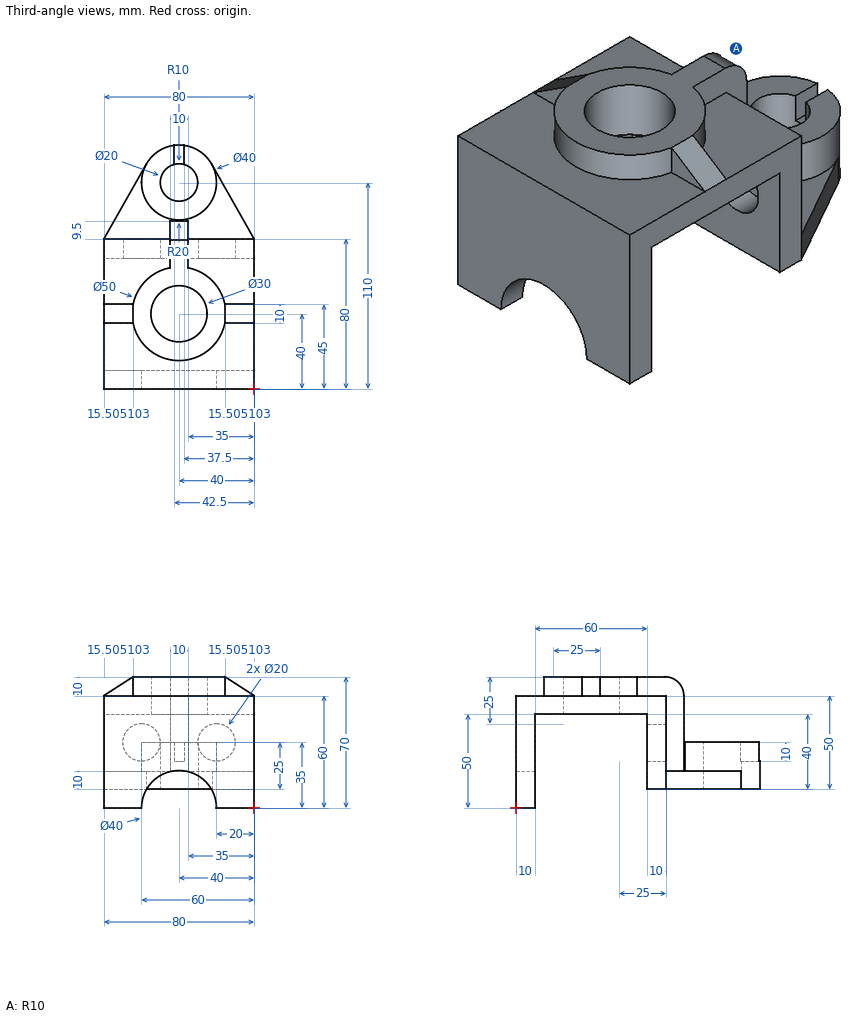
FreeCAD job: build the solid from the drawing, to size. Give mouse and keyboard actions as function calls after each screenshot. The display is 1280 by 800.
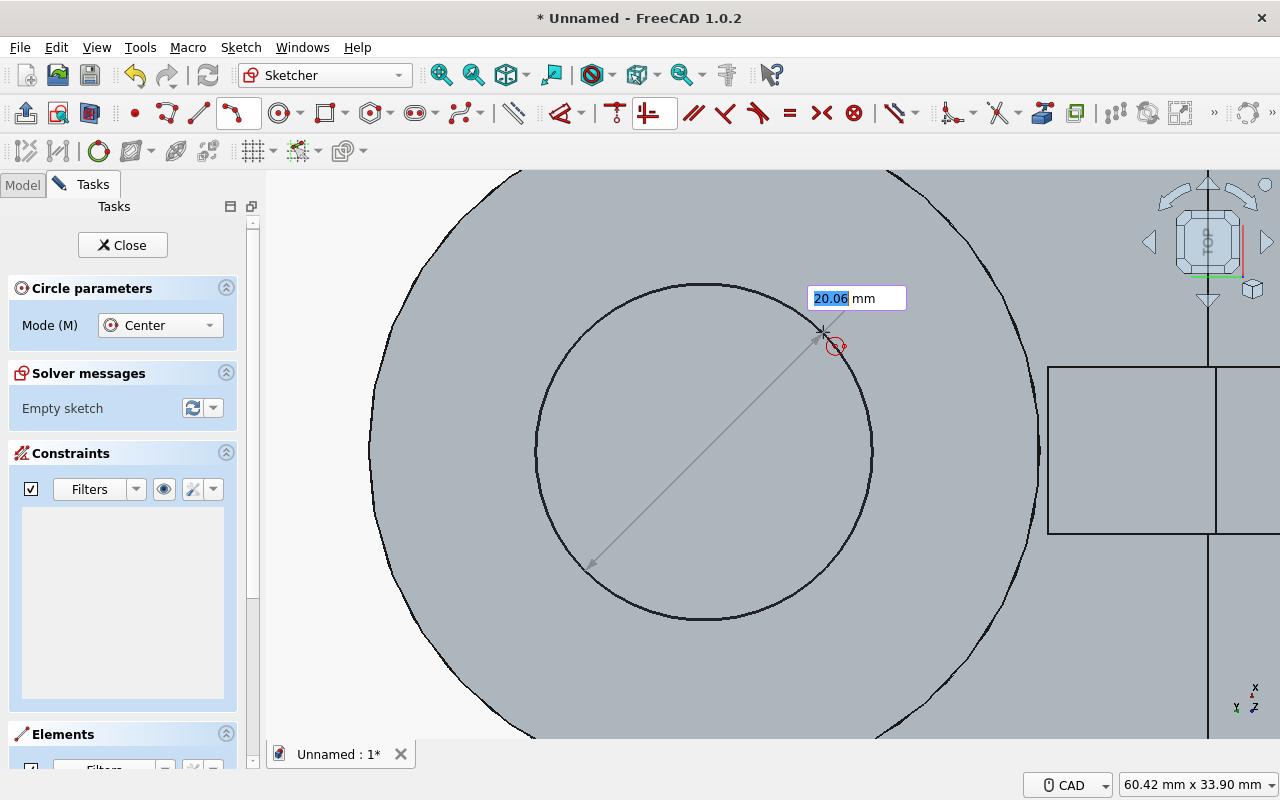
text(20)
key(Return)
key(Escape)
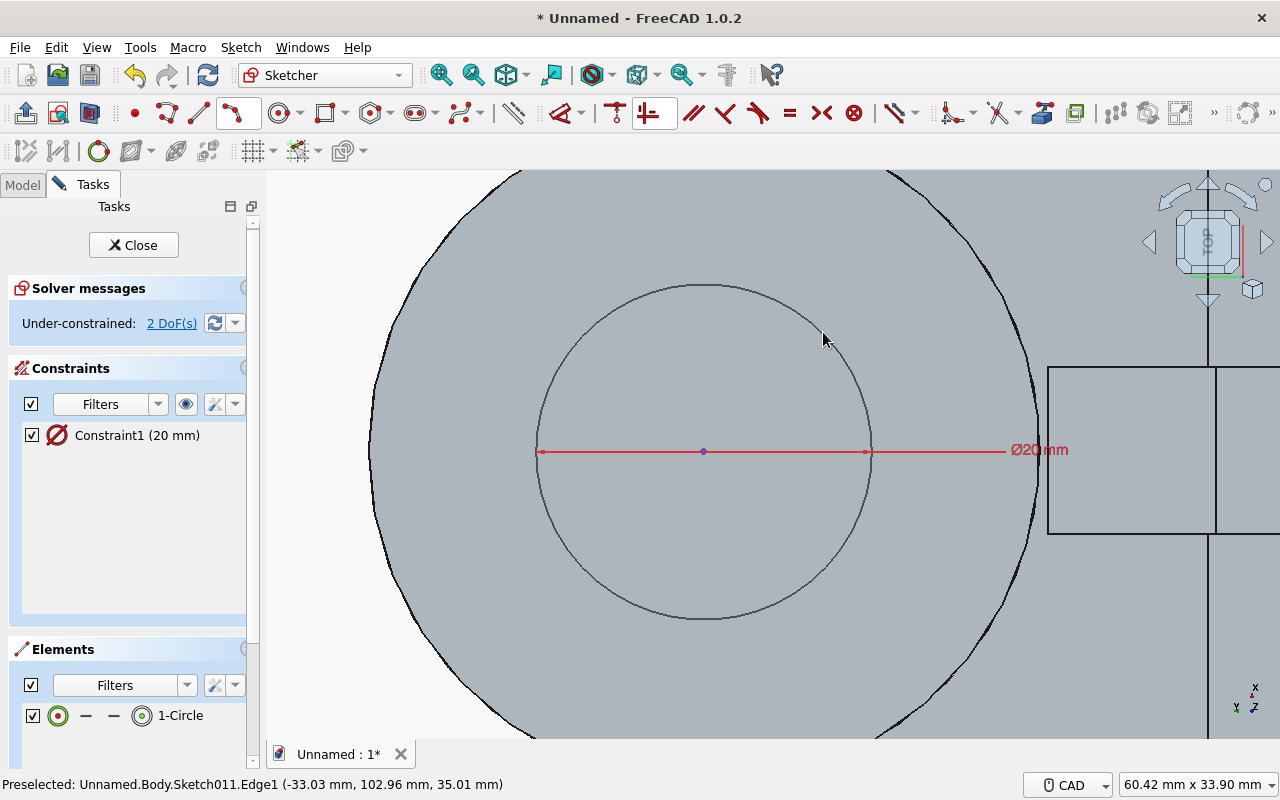
click(560, 114)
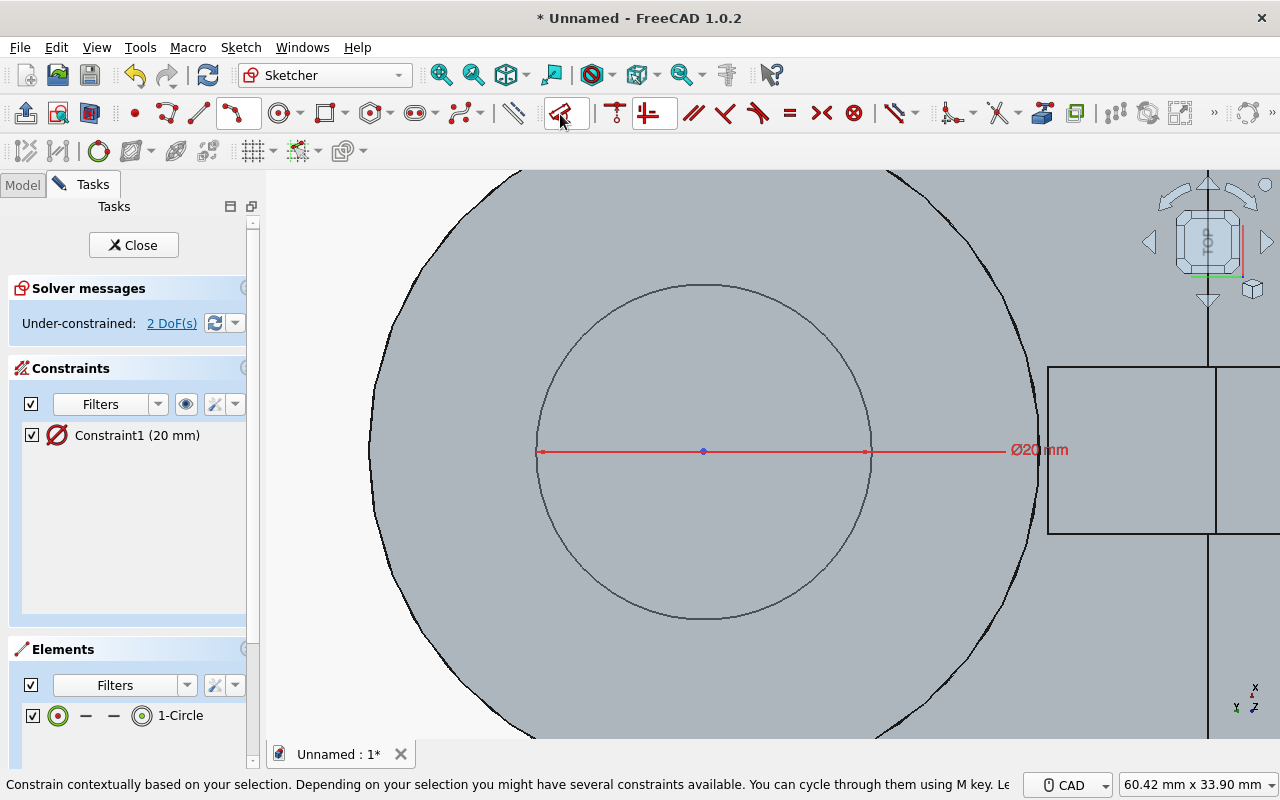
click(704, 452)
click(670, 325)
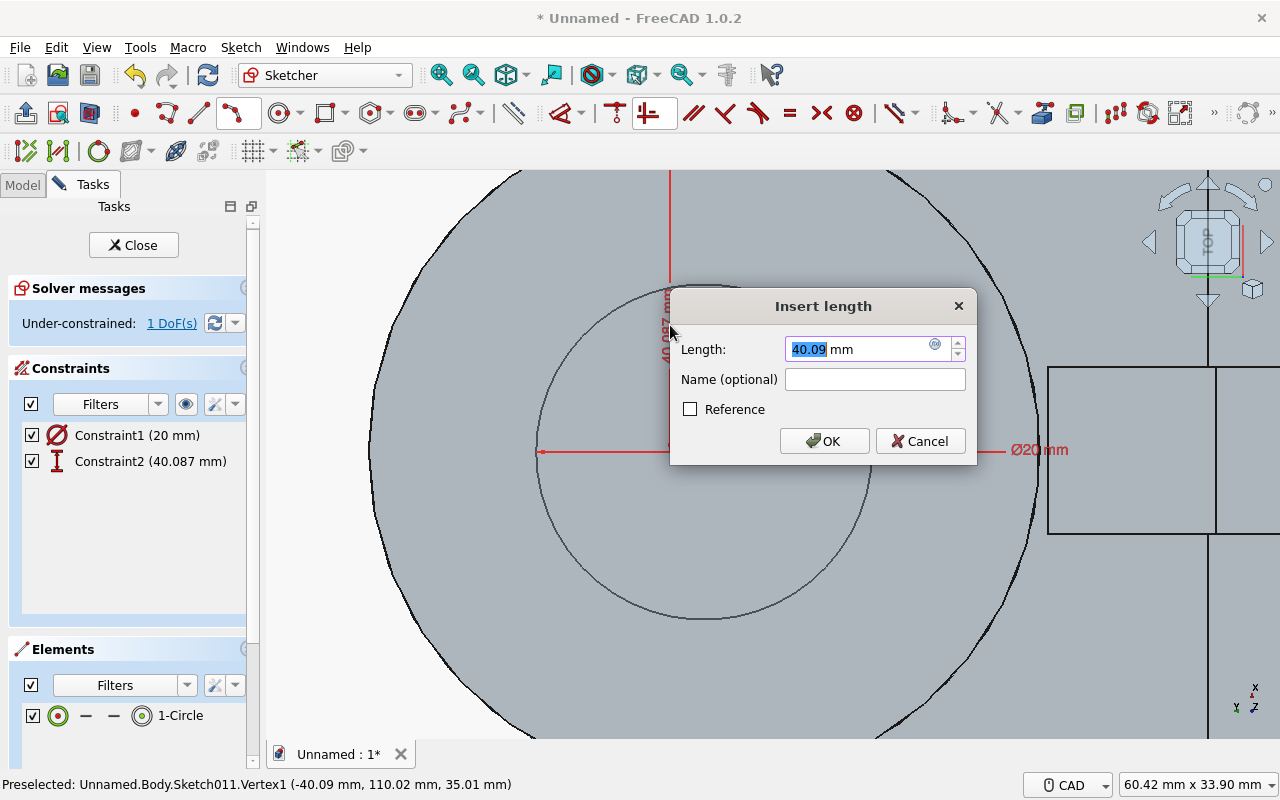
text(40)
key(Return)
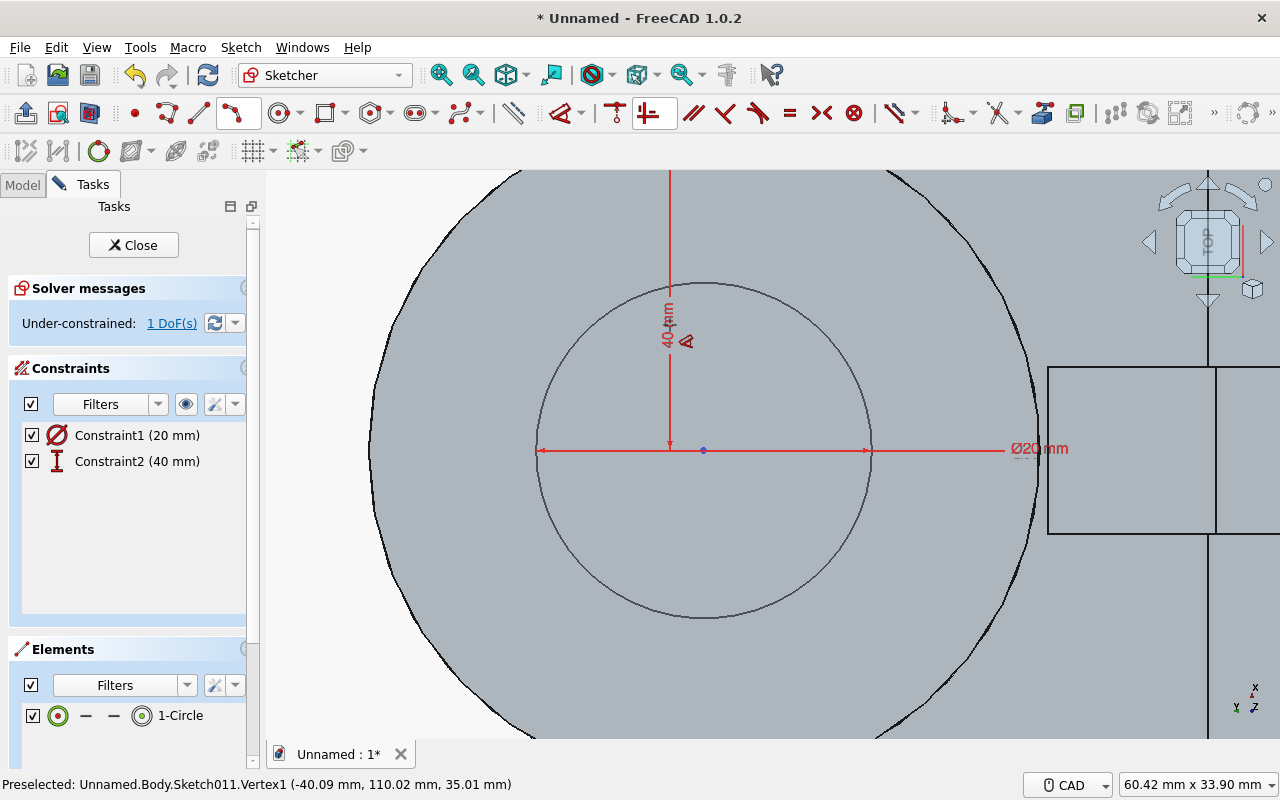
click(704, 451)
click(910, 485)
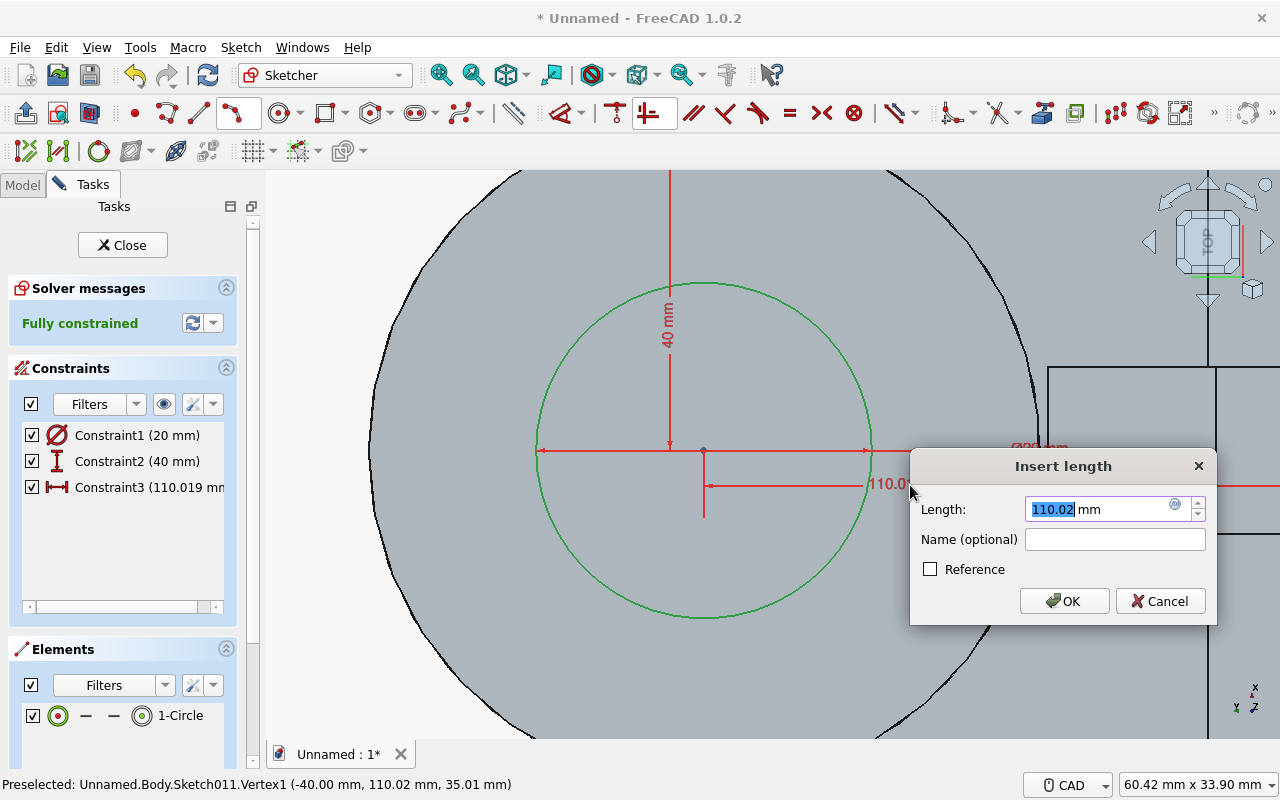
text(110)
key(Return)
key(Escape)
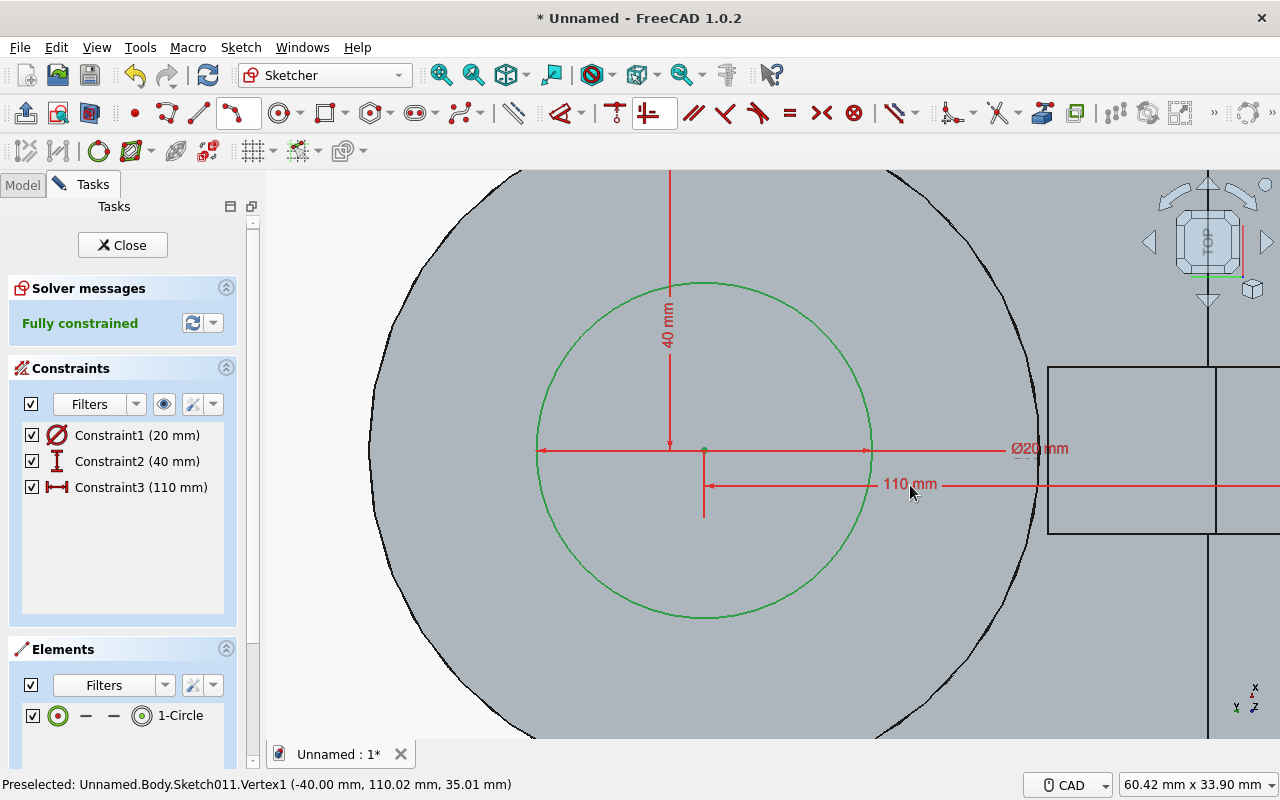
click(123, 245)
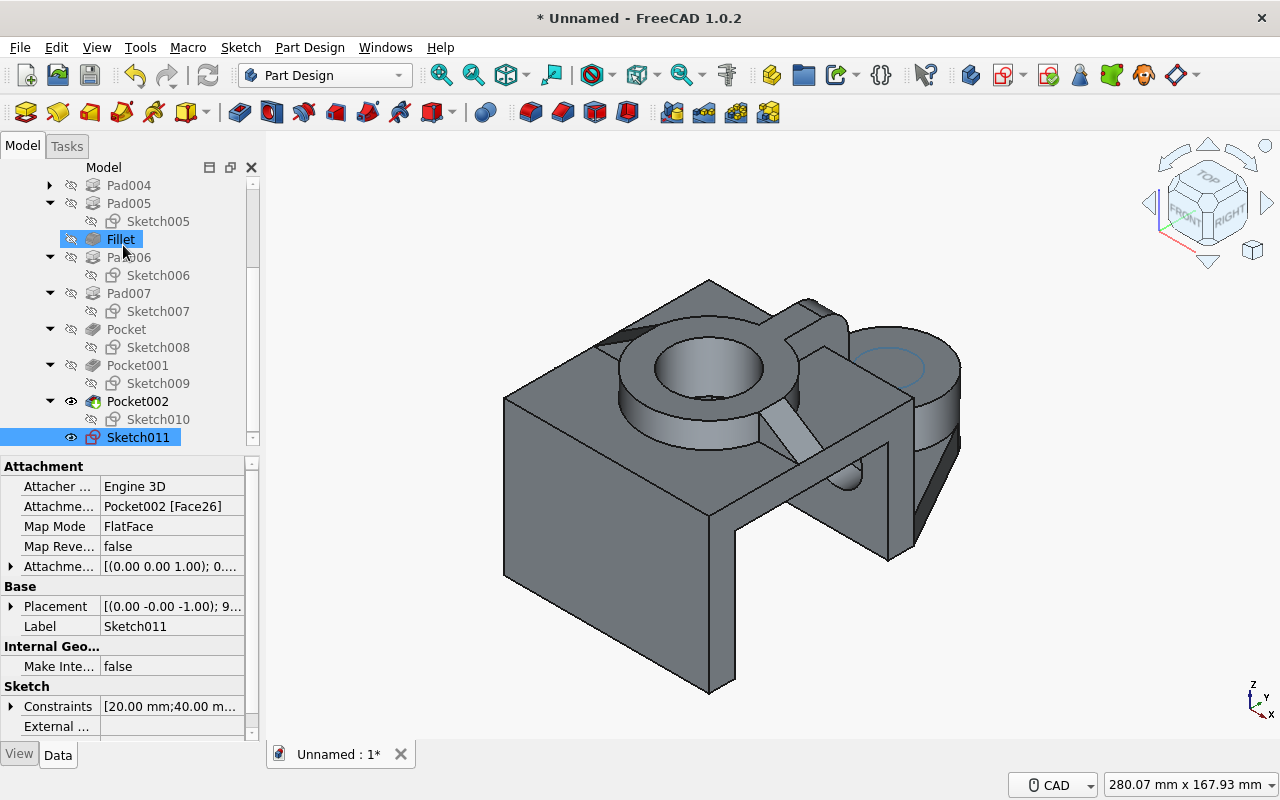
click(240, 112)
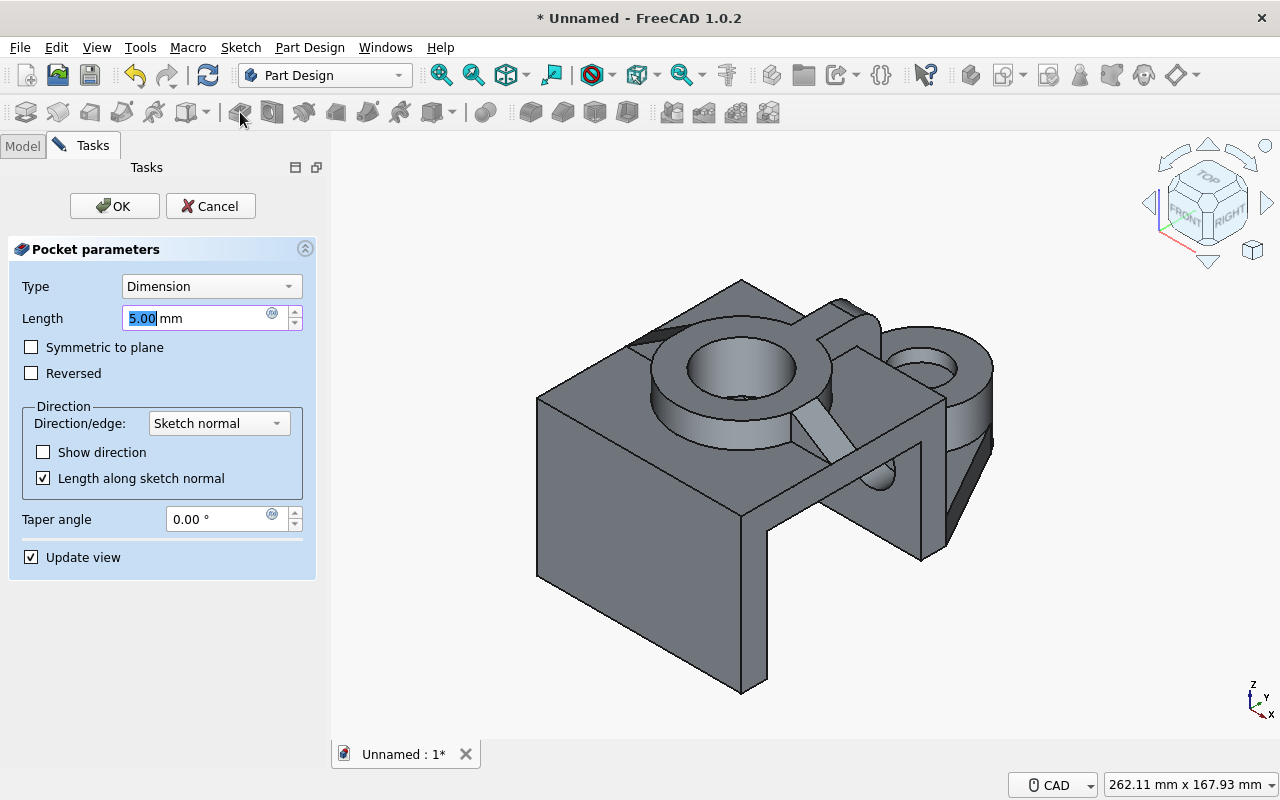
click(212, 286)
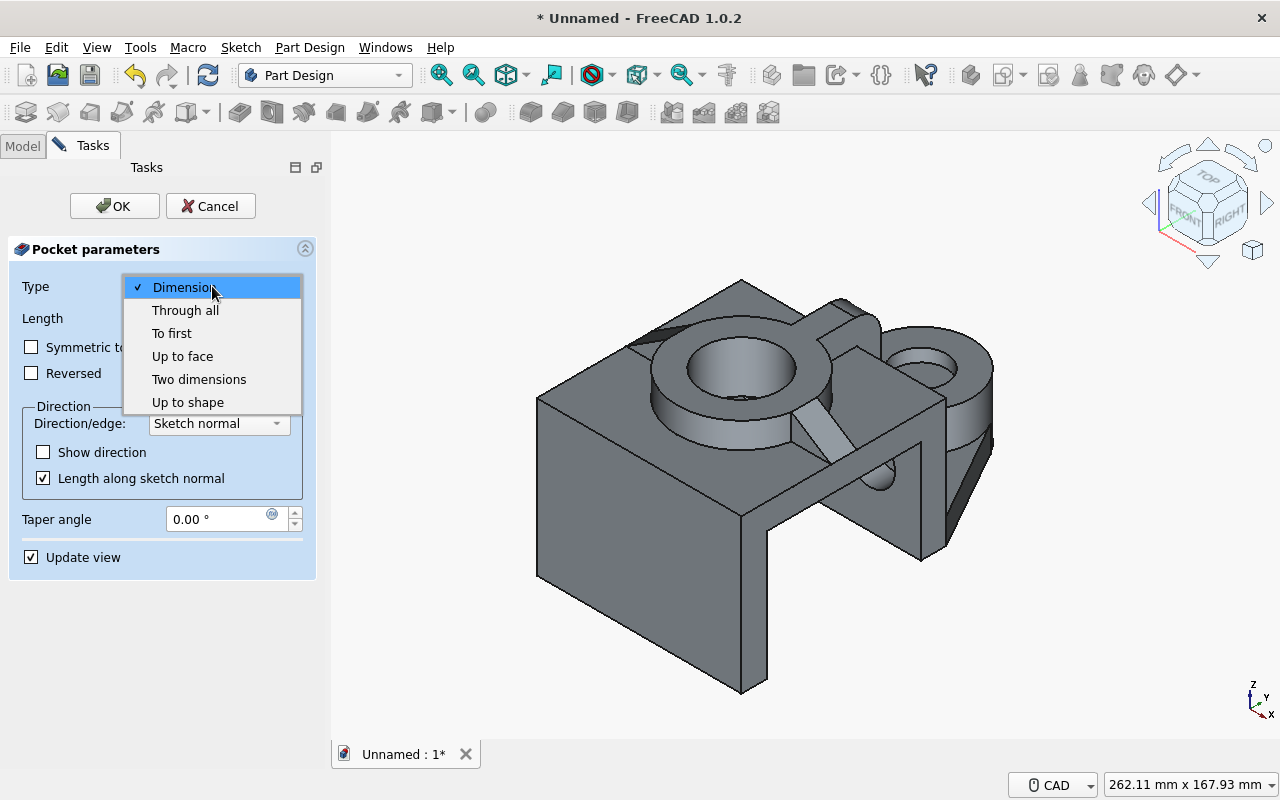
click(212, 310)